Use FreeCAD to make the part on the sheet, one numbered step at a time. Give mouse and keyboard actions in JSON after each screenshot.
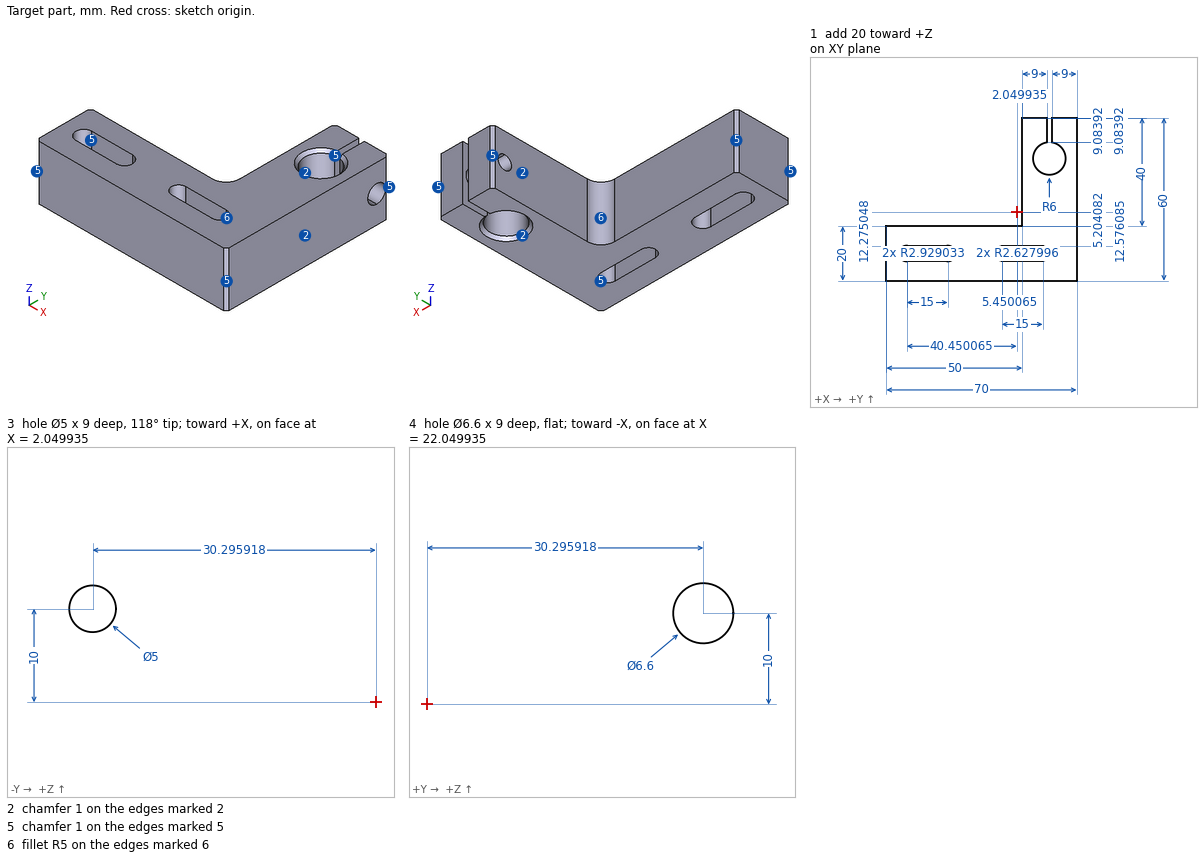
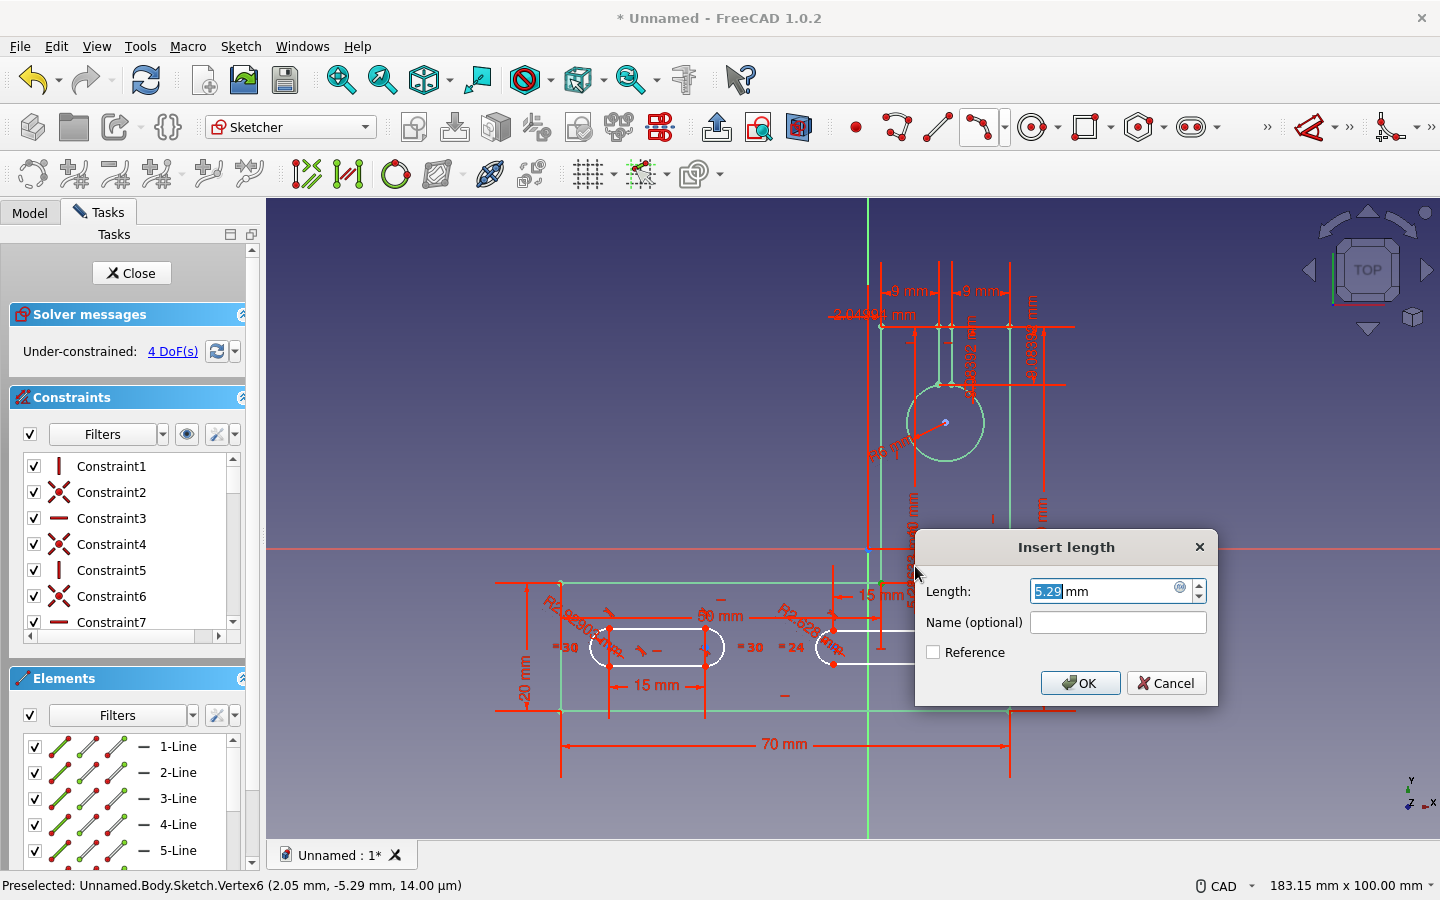
{"action": "type", "text": "5.204082"}
{"action": "key", "text": "Return"}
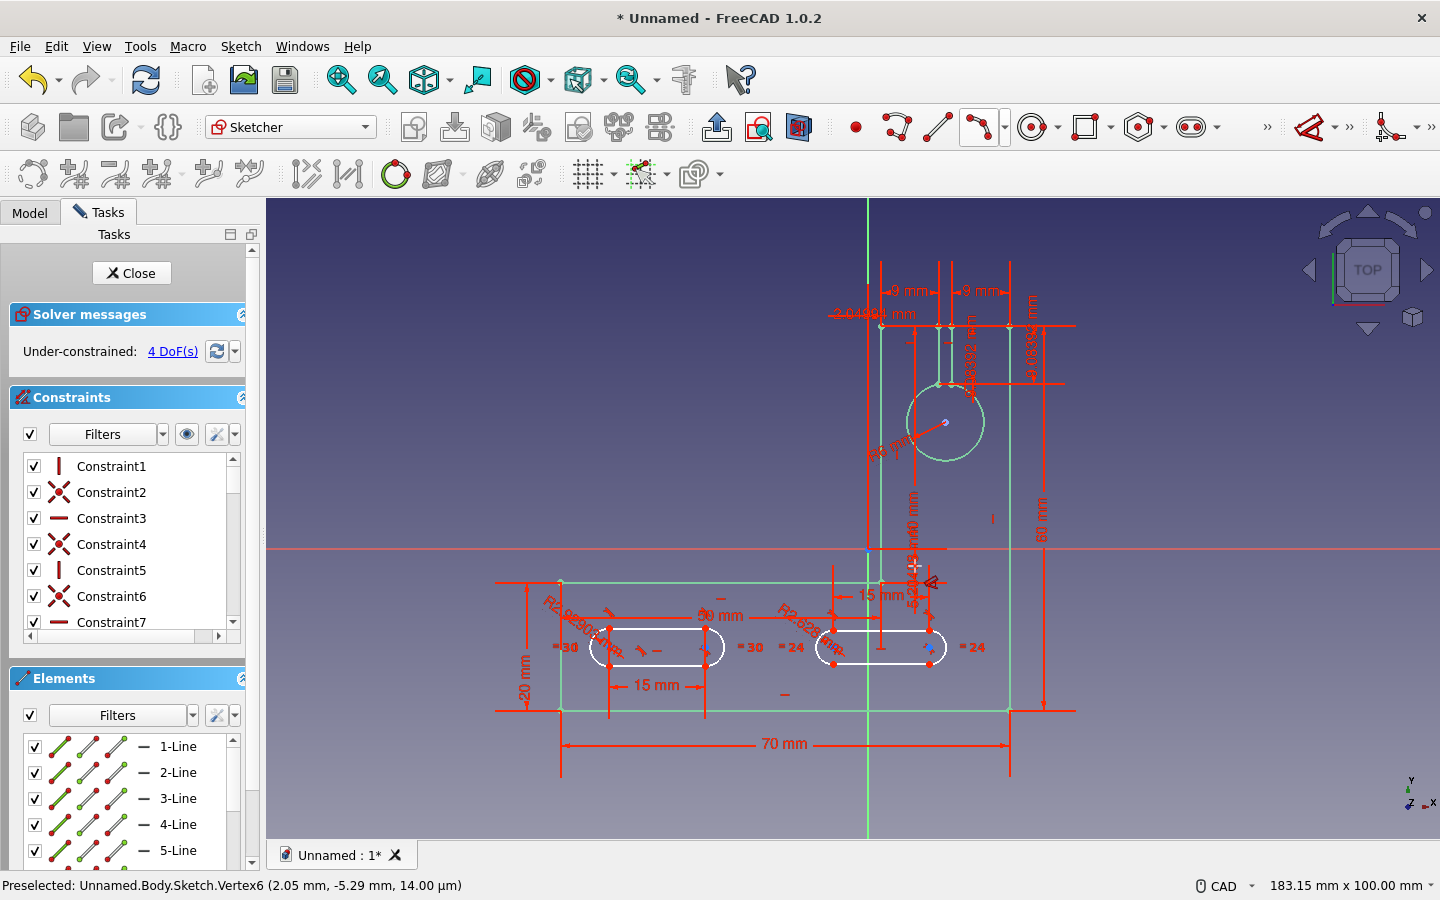
{"action": "left_click", "coordinate": [833, 631]}
{"action": "left_click", "coordinate": [843, 515]}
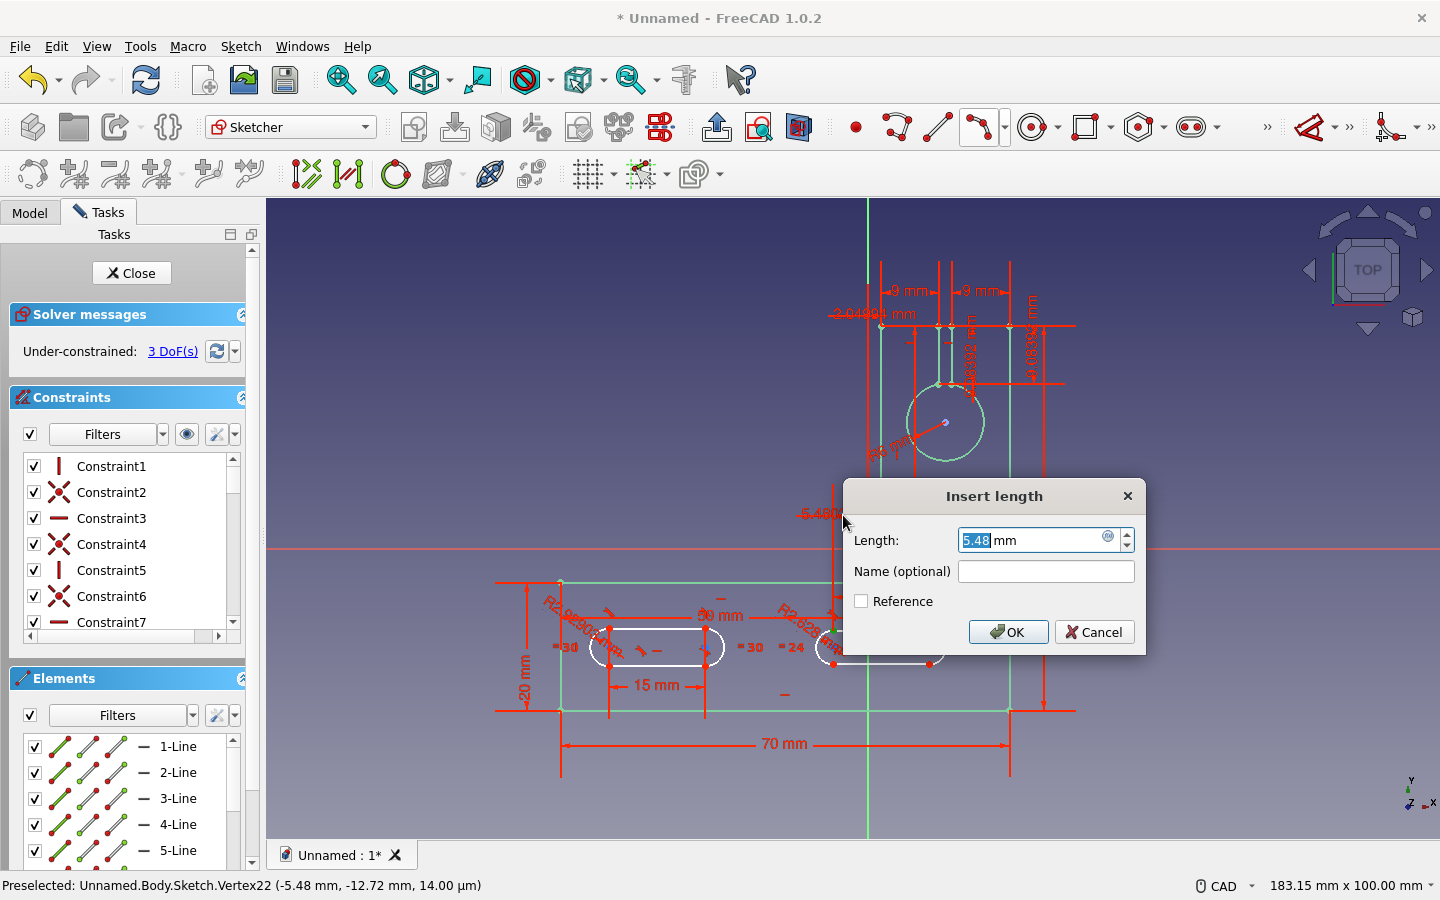
{"action": "type", "text": "5.450065"}
{"action": "key", "text": "Return"}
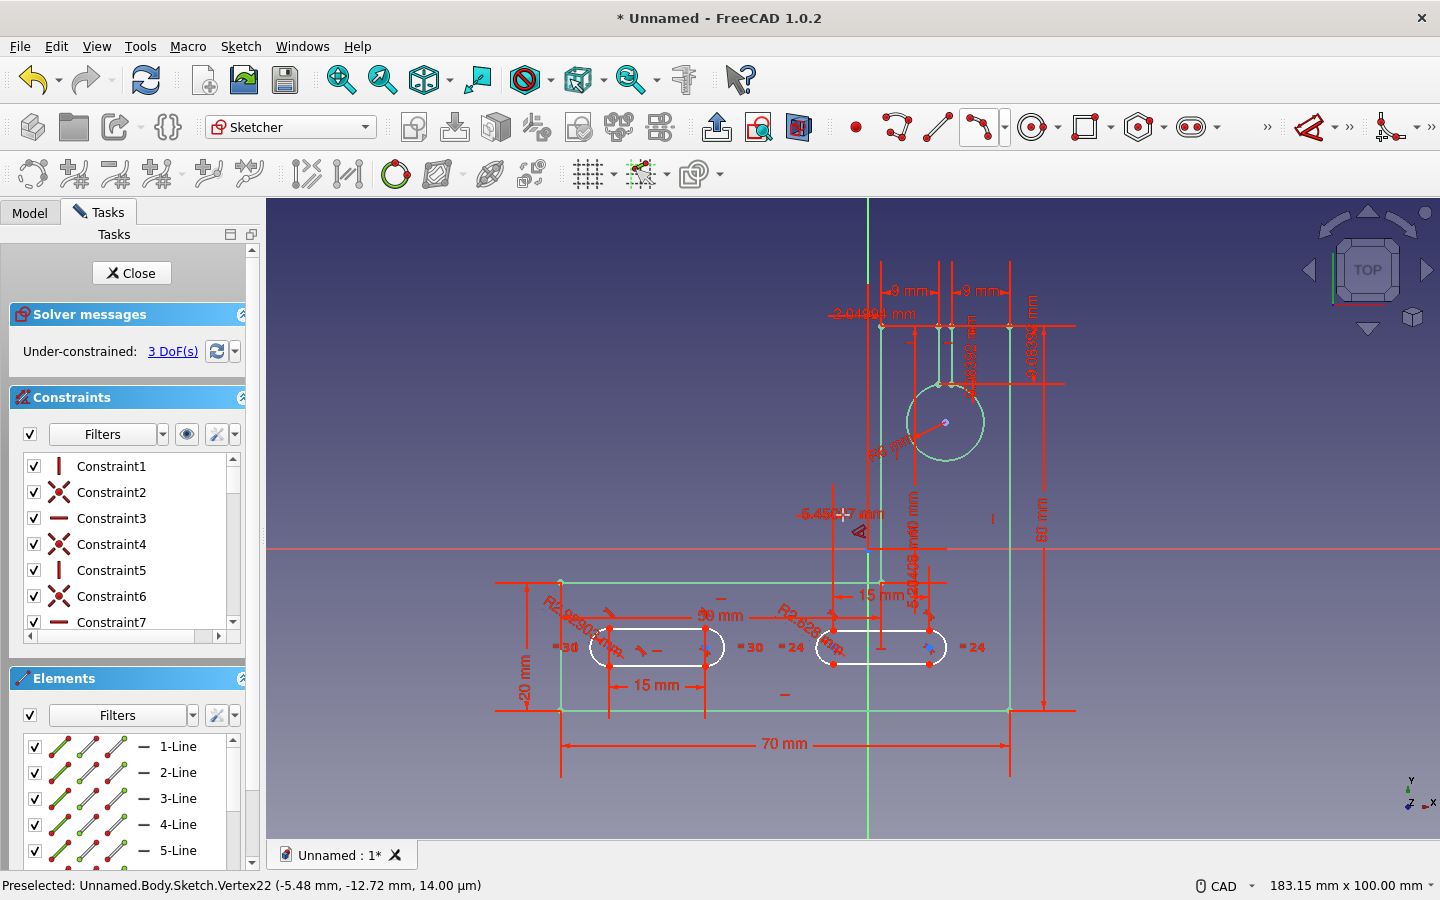
{"action": "left_click", "coordinate": [833, 631]}
{"action": "left_click", "coordinate": [799, 609]}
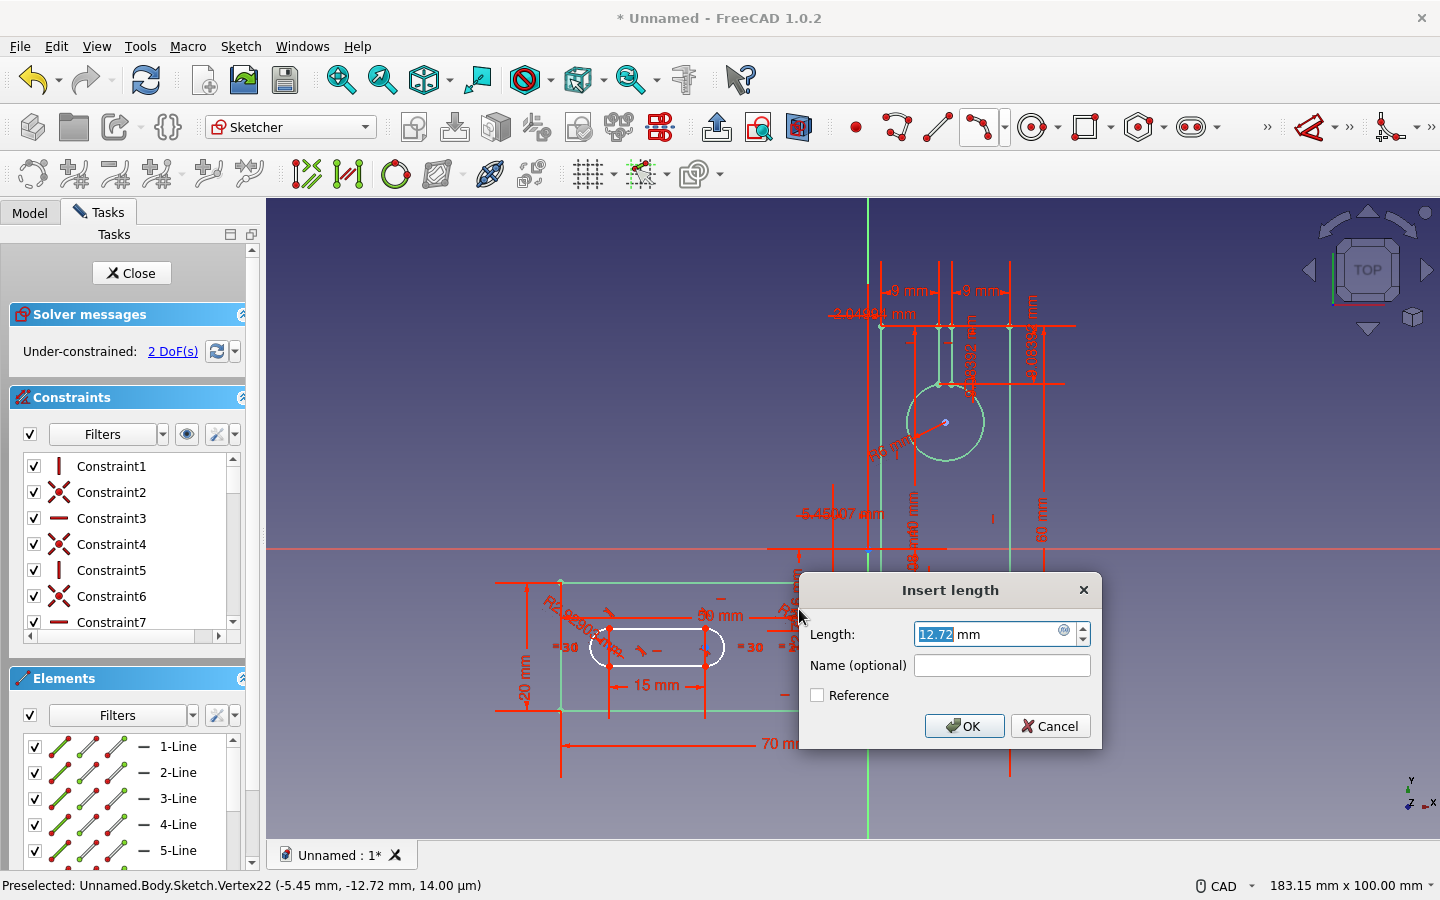
{"action": "type", "text": "12.576085"}
{"action": "key", "text": "Return"}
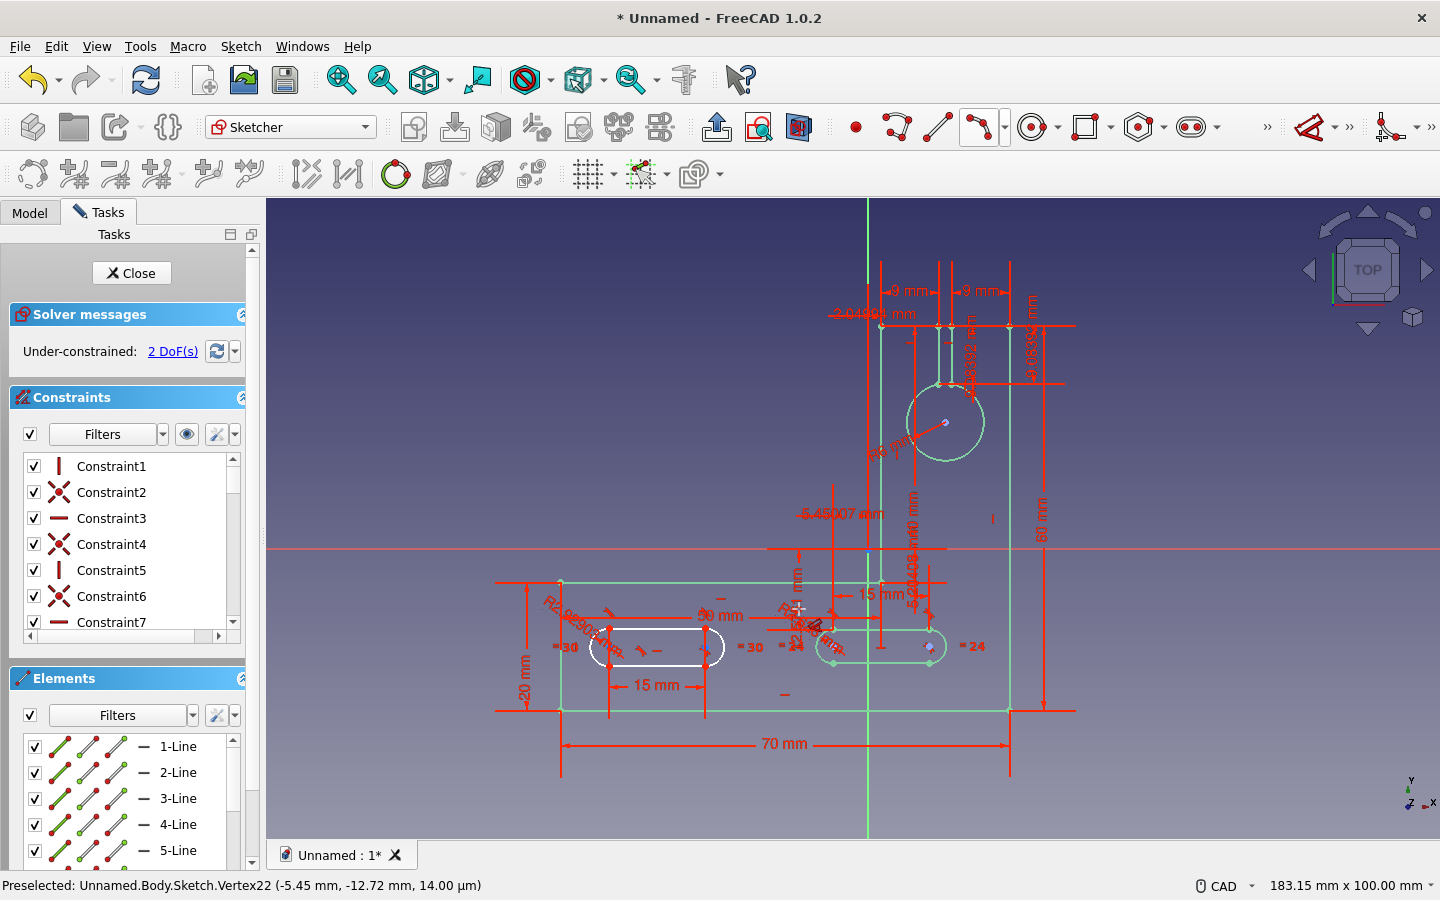
{"action": "left_click", "coordinate": [609, 629]}
{"action": "left_click", "coordinate": [739, 663]}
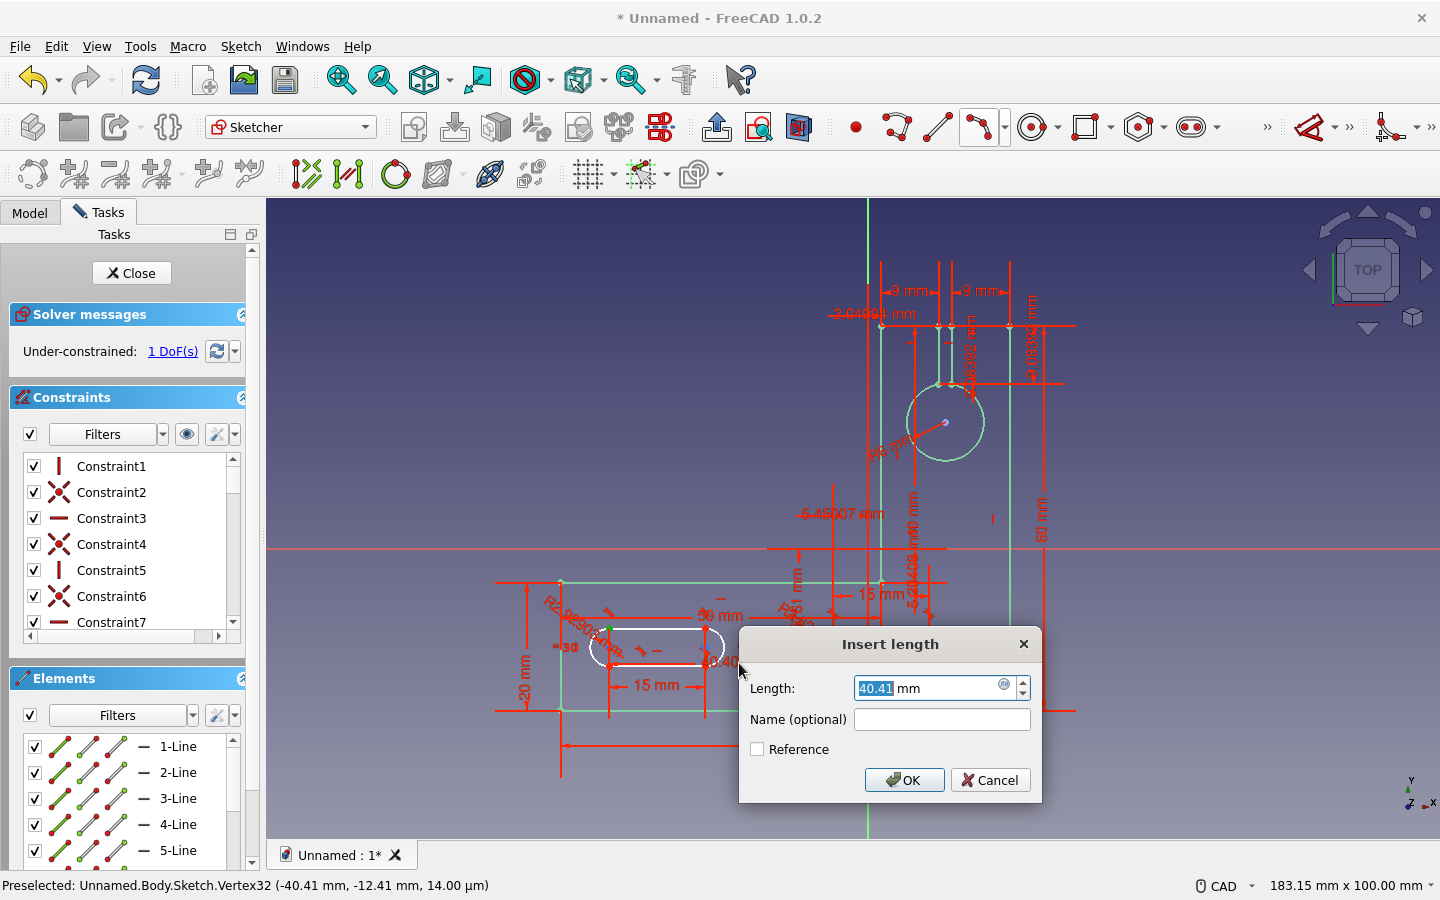
{"action": "type", "text": "40.450065"}
{"action": "key", "text": "Return"}